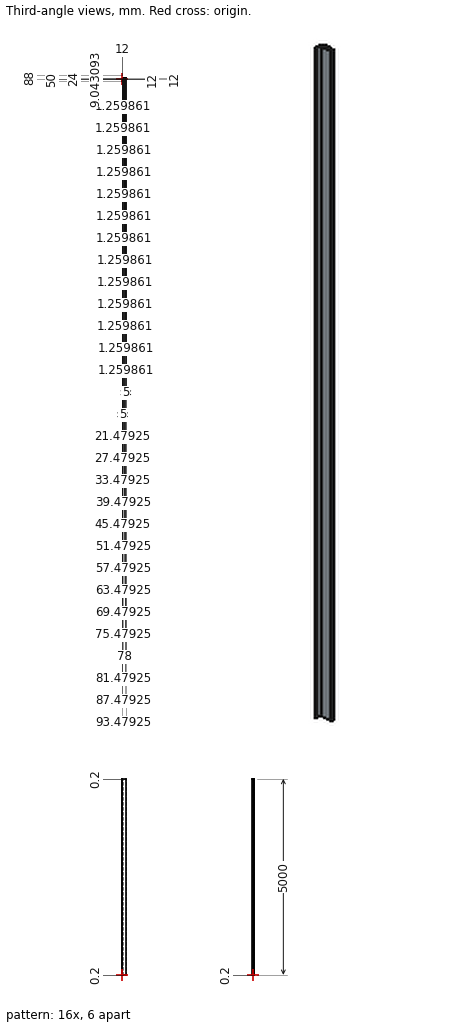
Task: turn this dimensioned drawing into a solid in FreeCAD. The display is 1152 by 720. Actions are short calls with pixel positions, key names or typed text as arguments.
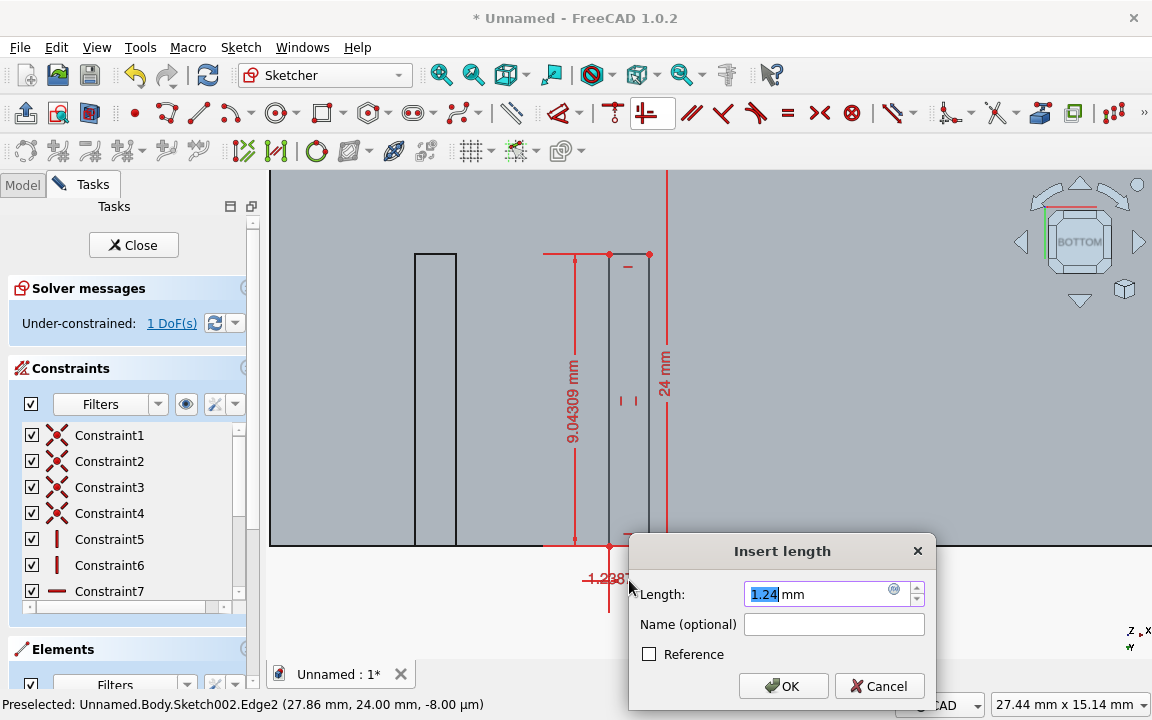
text(1.259861)
key(Return)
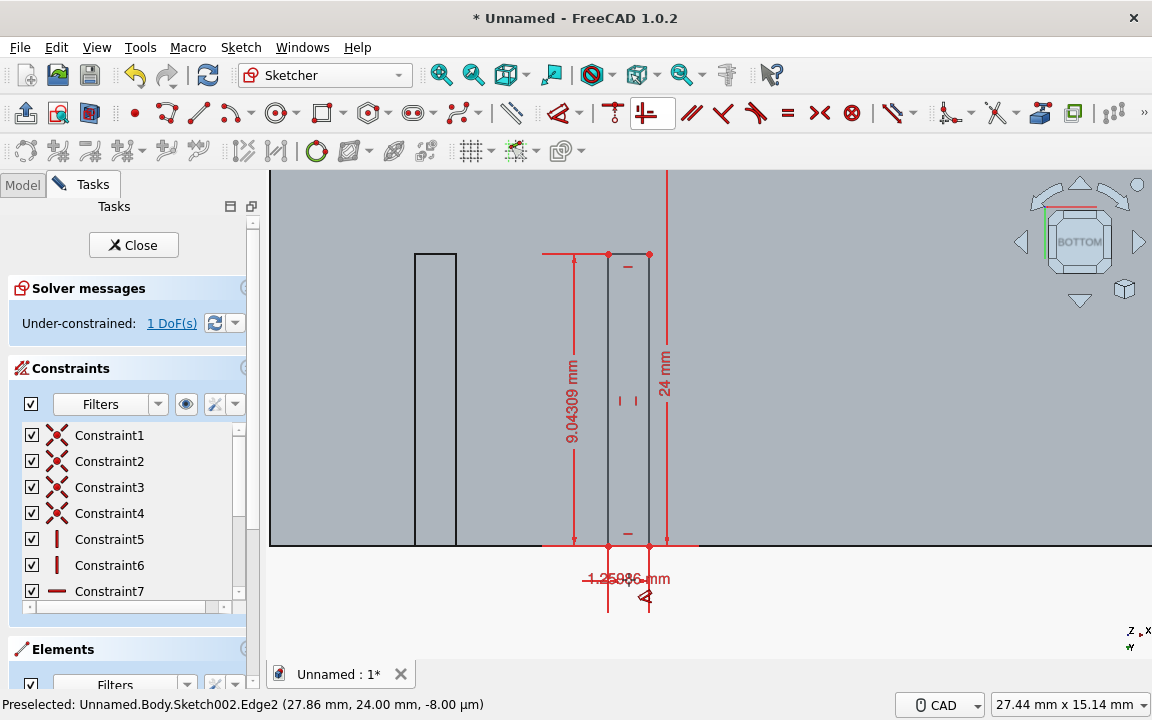
click(608, 254)
click(451, 288)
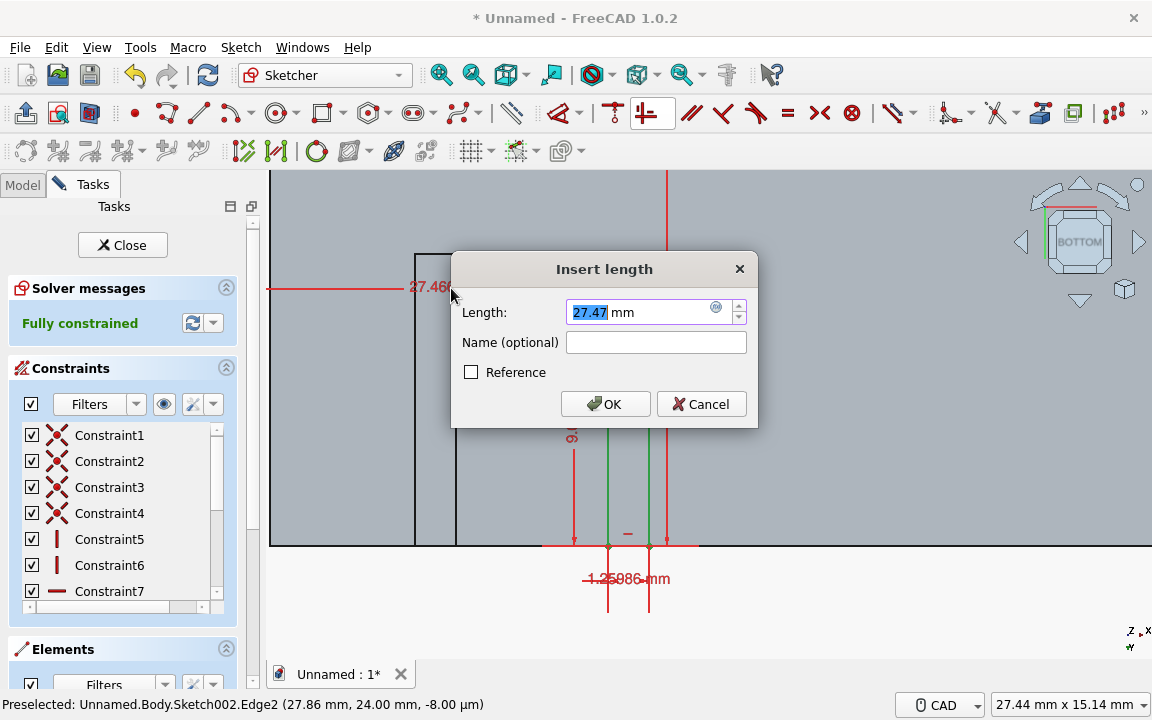
text(27.47925)
key(Return)
key(Escape)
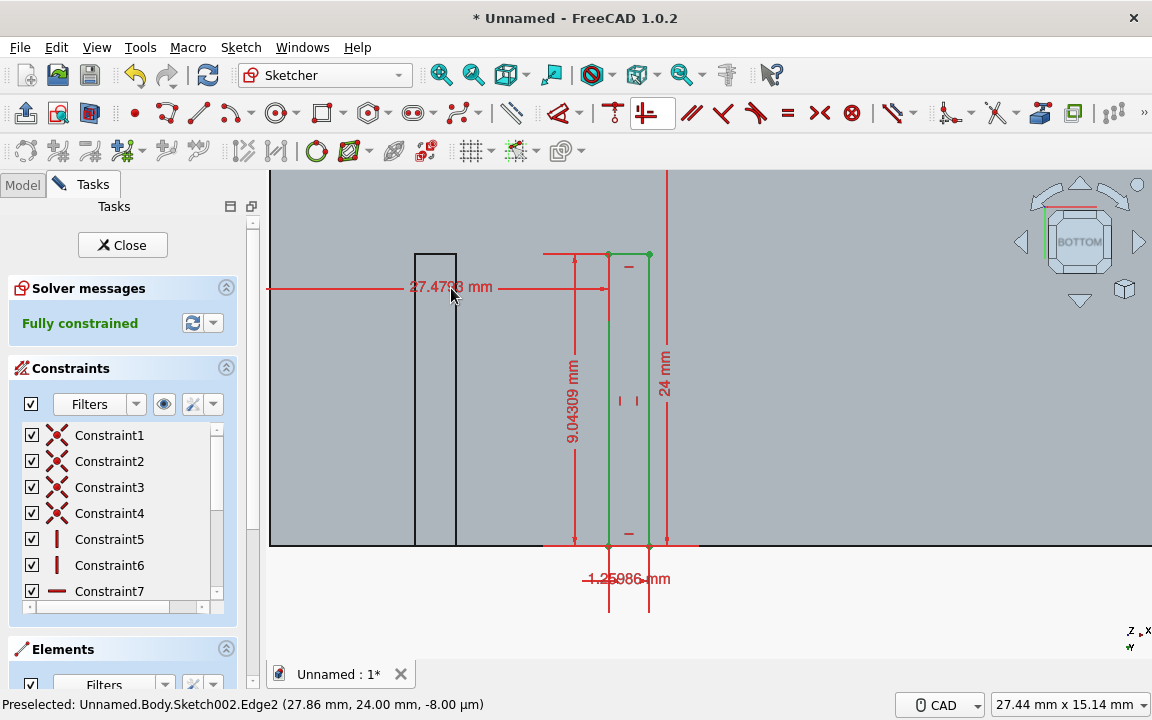
click(123, 245)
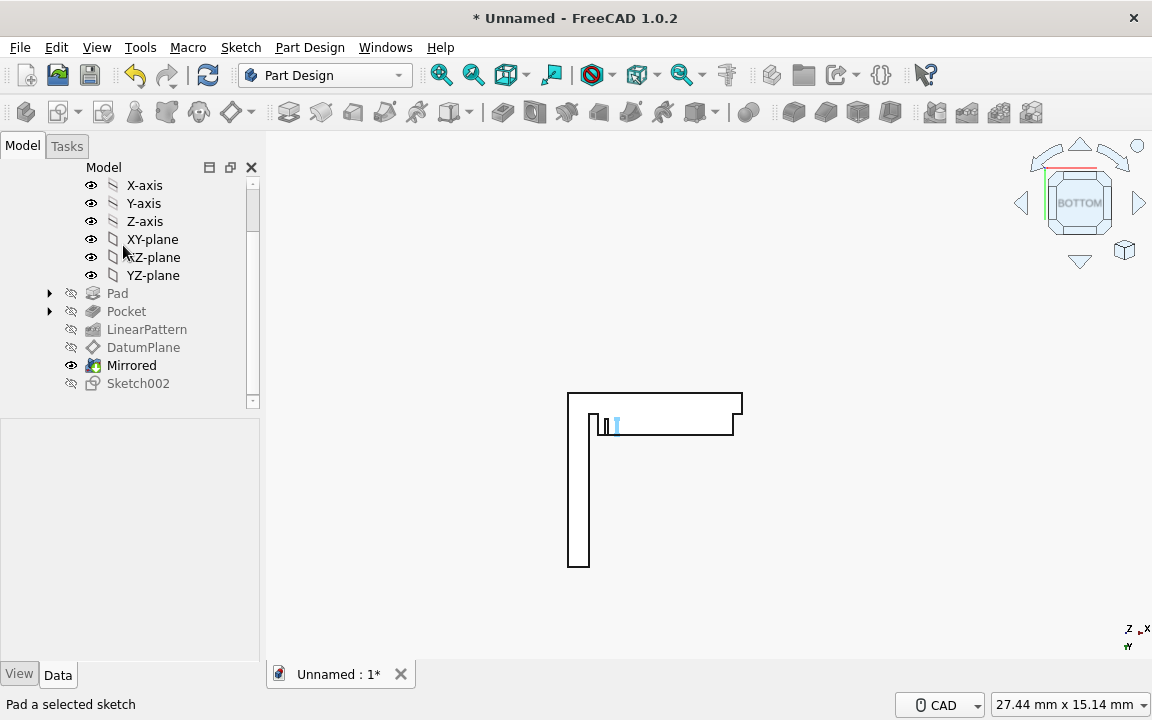
click(504, 112)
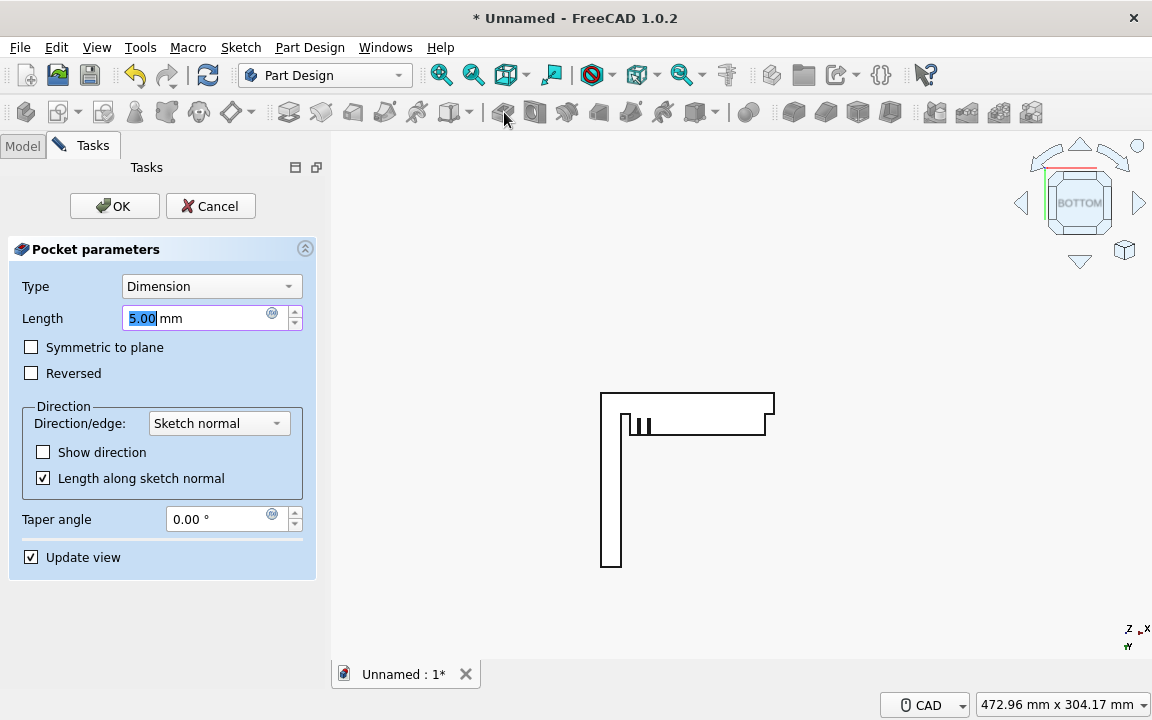
text(0.2)
key(Tab)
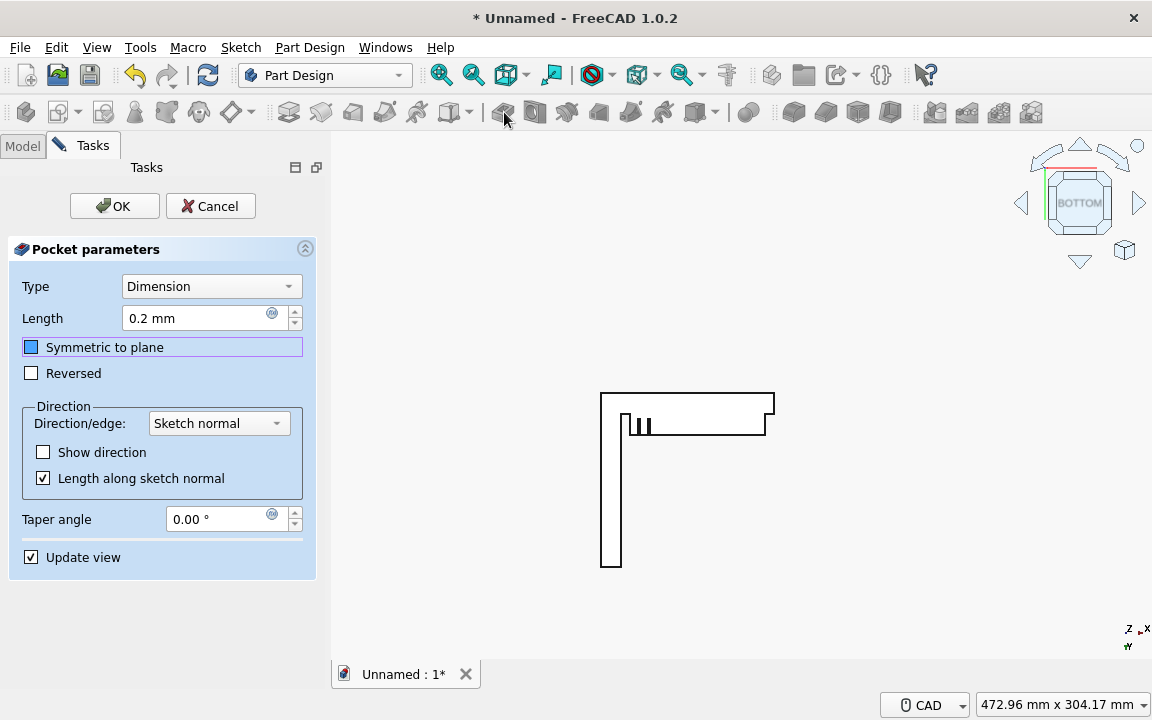
click(115, 206)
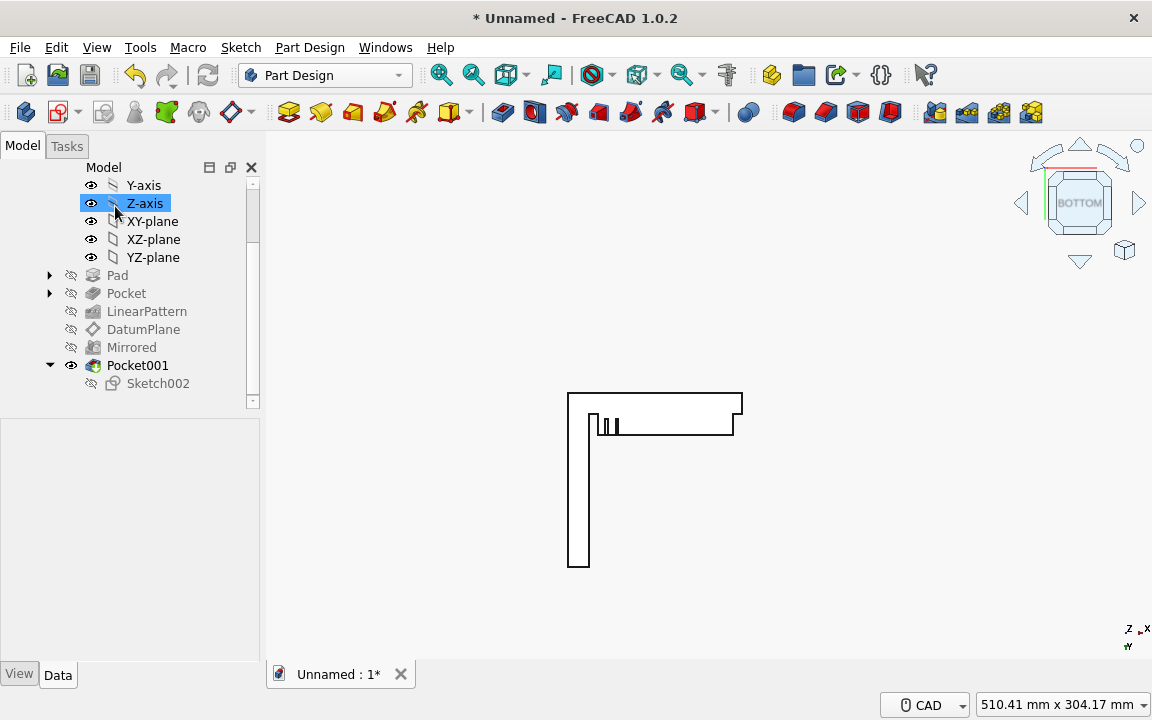
key(v)
key(f)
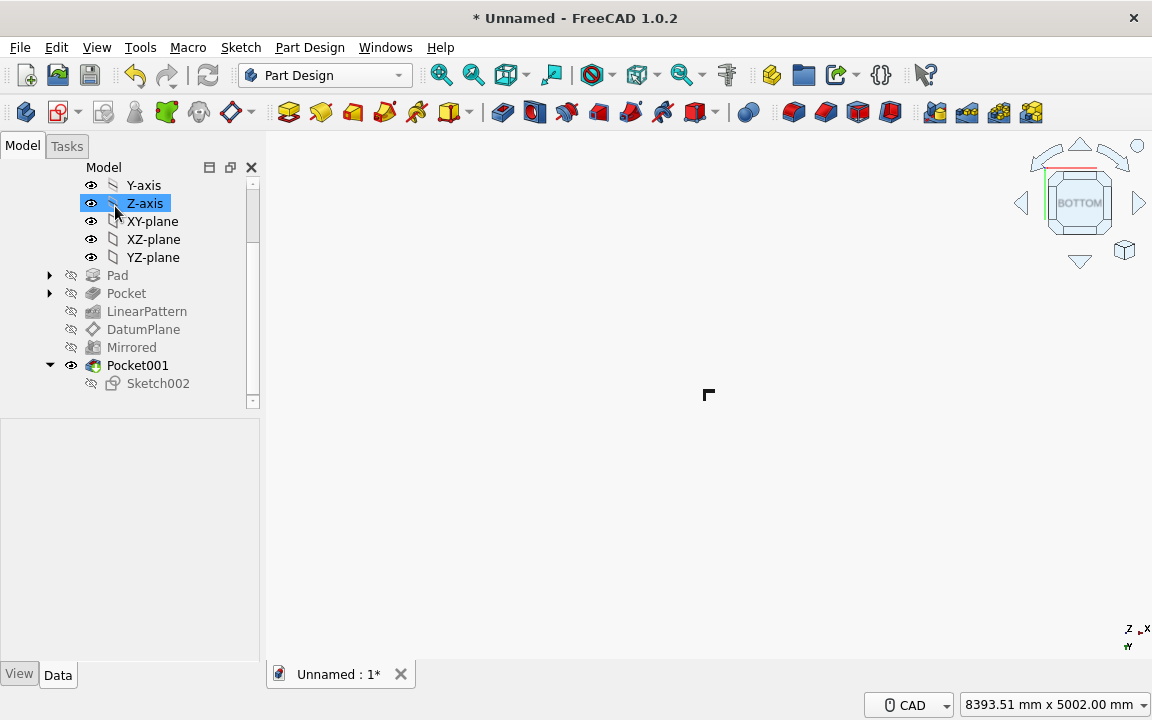
click(58, 112)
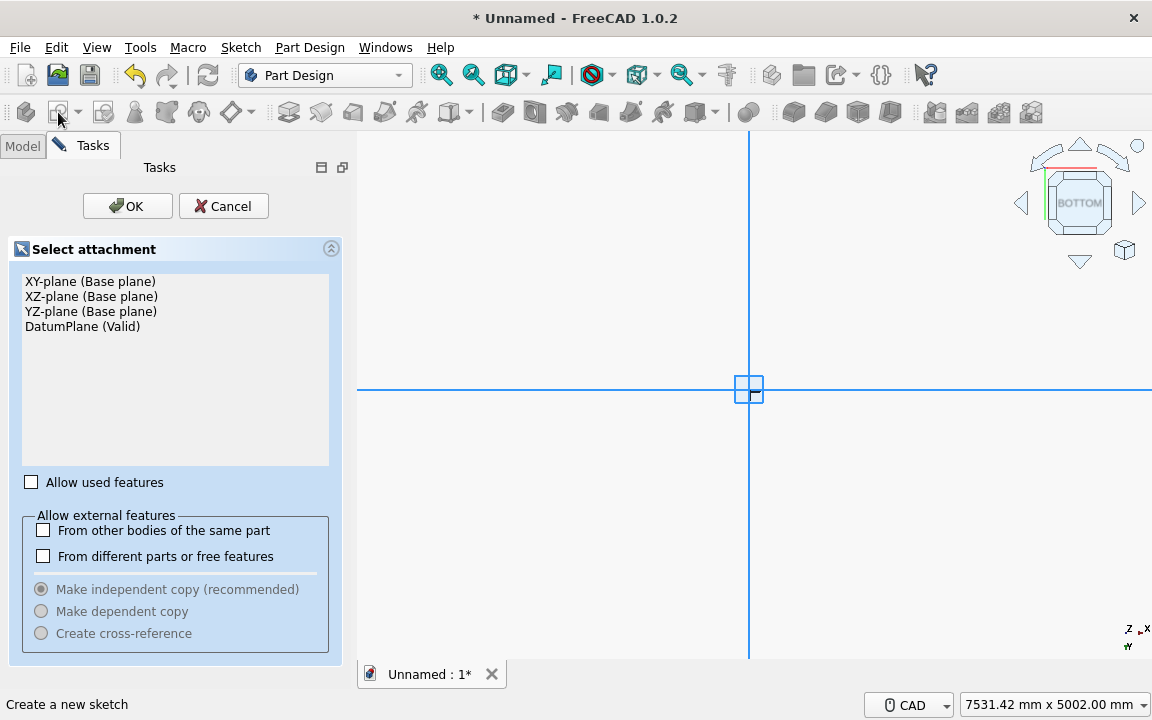
click(82, 282)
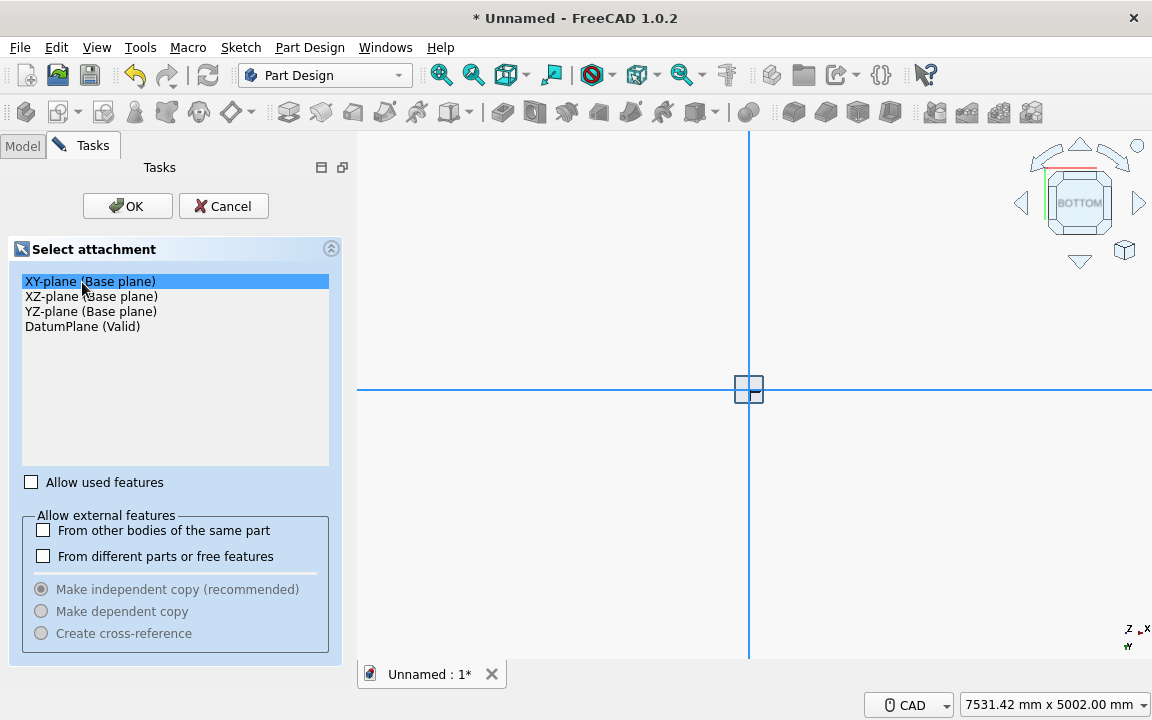
click(128, 206)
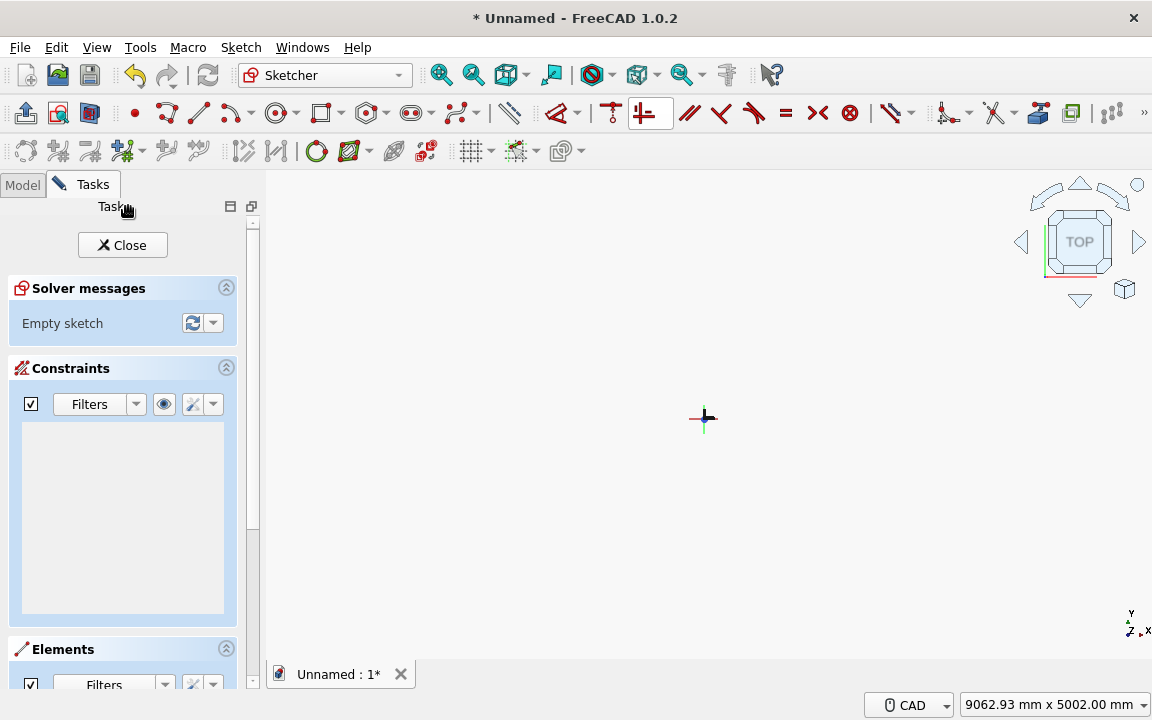
click(90, 114)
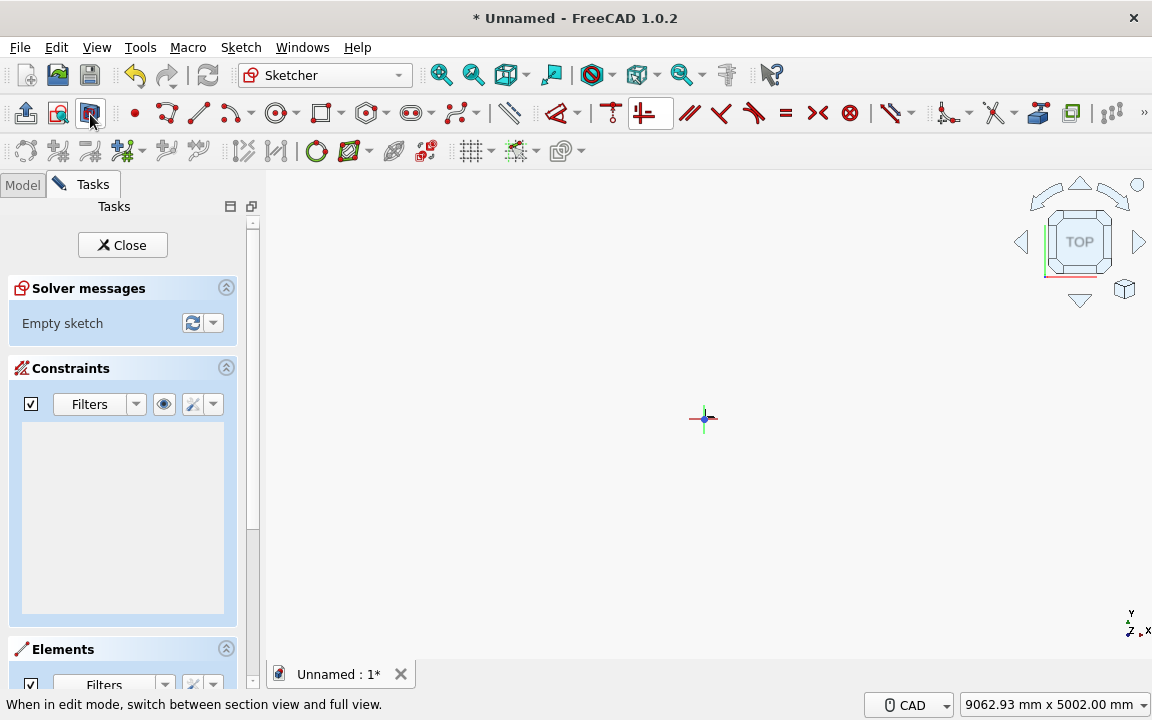
scroll(711, 418, up, 15)